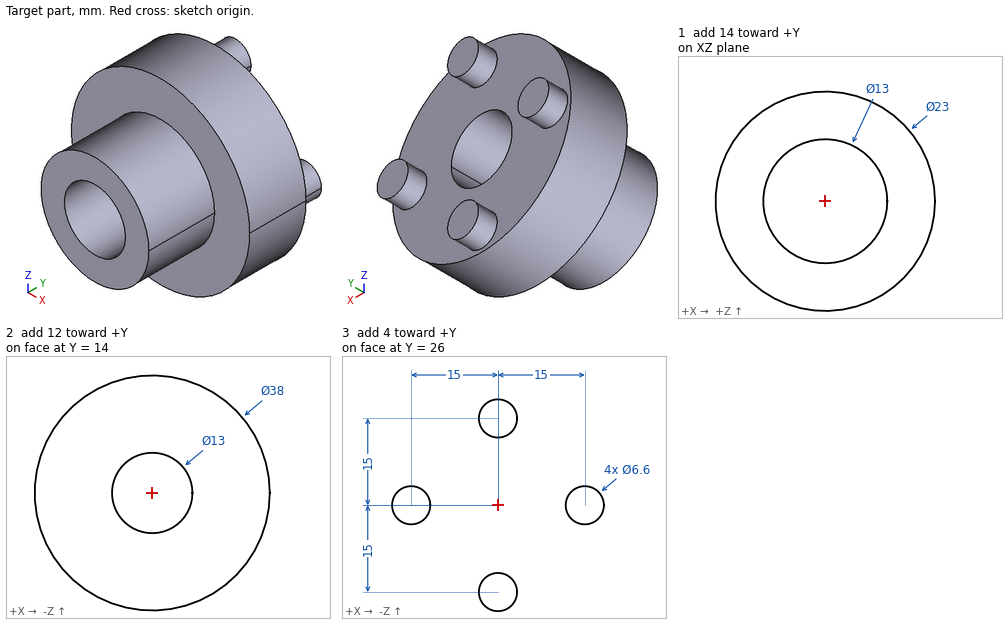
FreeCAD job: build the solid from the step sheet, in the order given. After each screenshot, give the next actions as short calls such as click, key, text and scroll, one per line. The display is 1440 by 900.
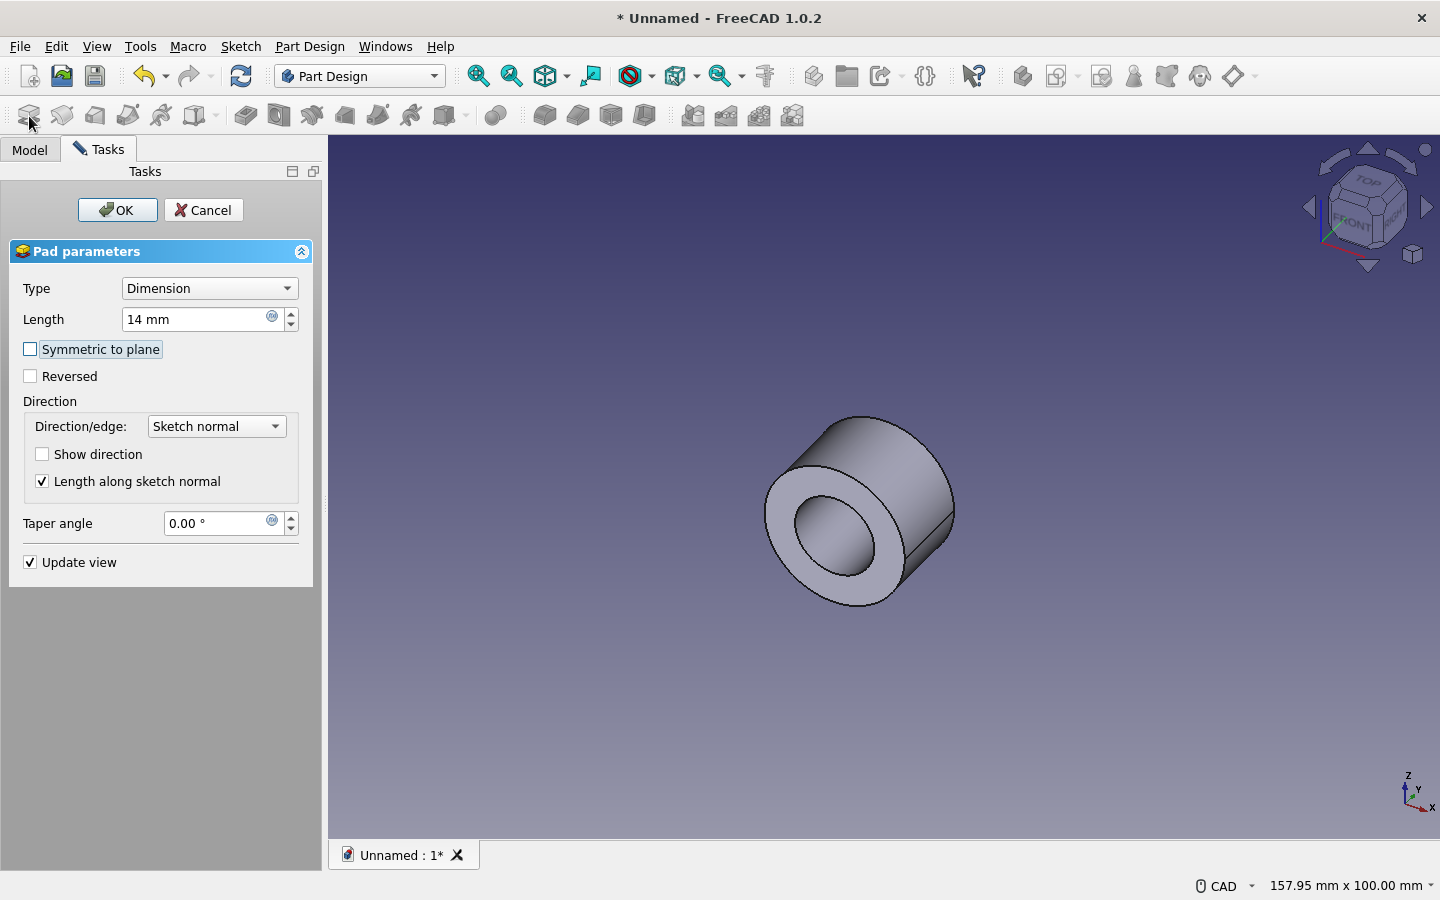
click(31, 376)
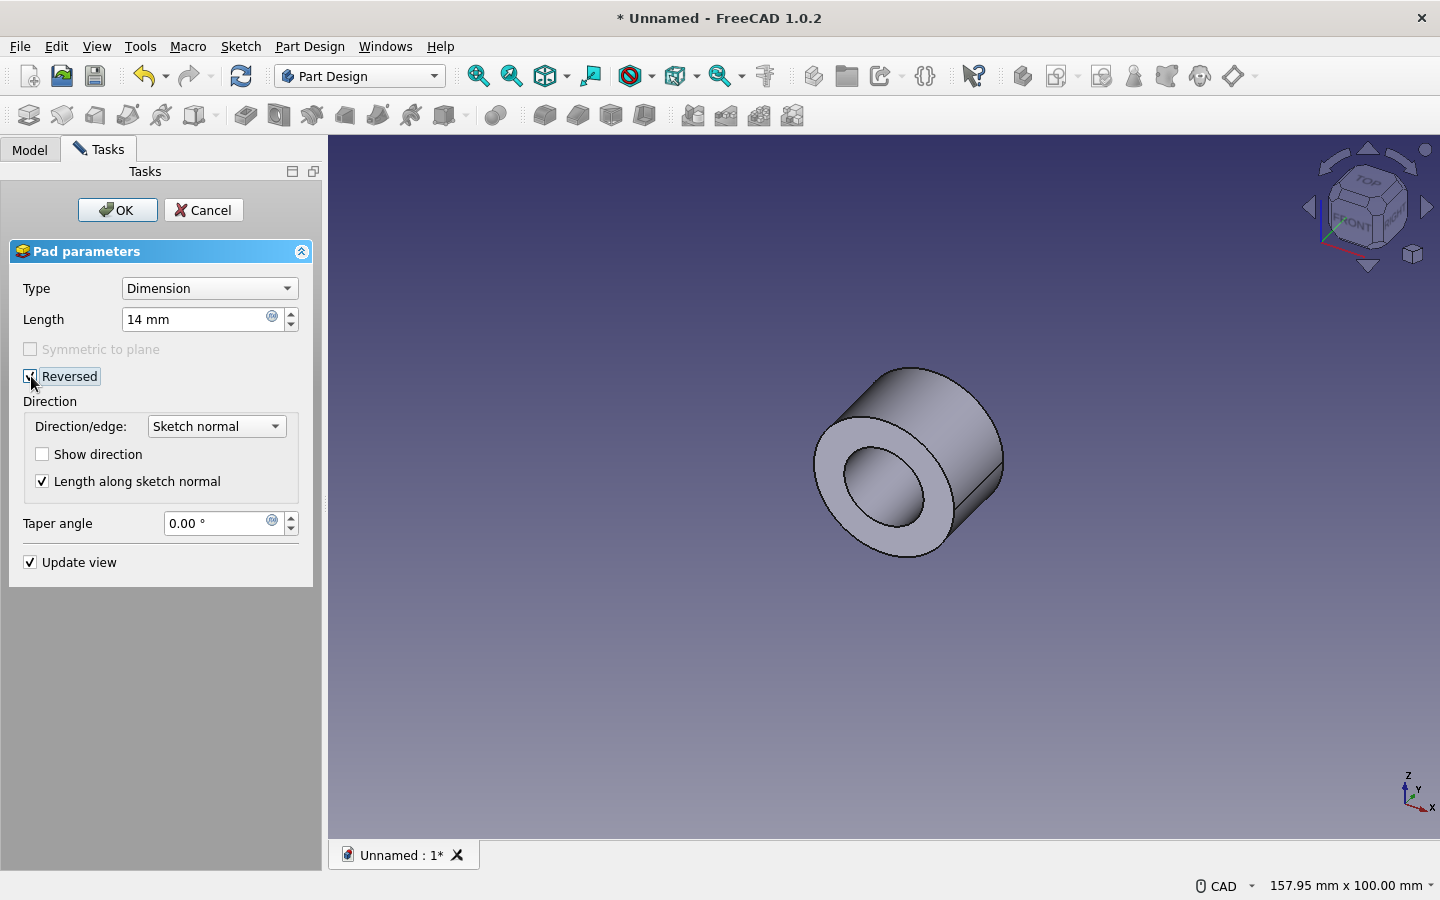
click(118, 210)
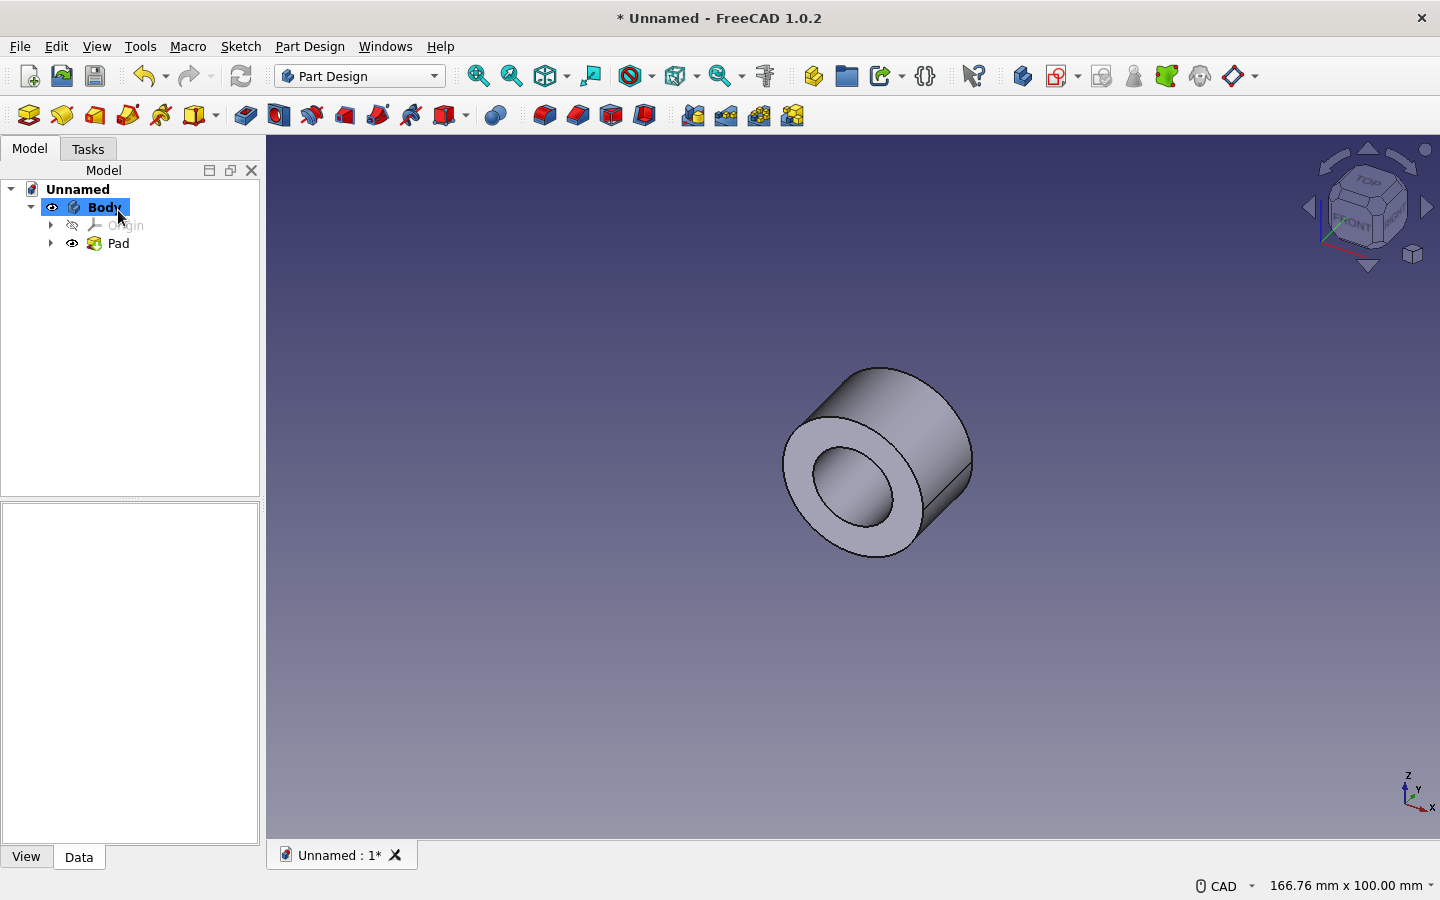
key(v)
key(f)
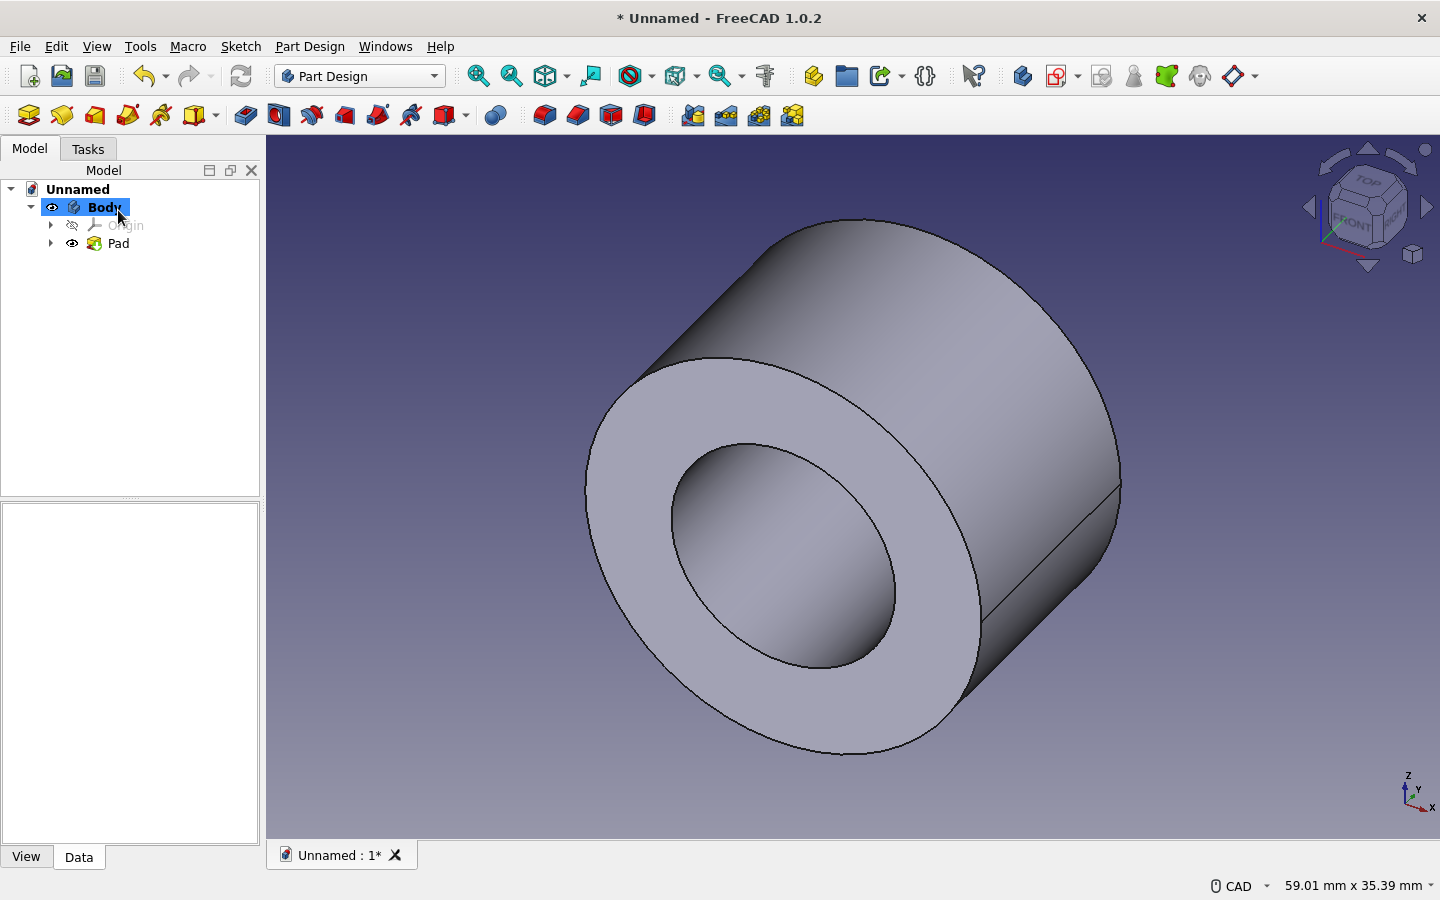
key(4)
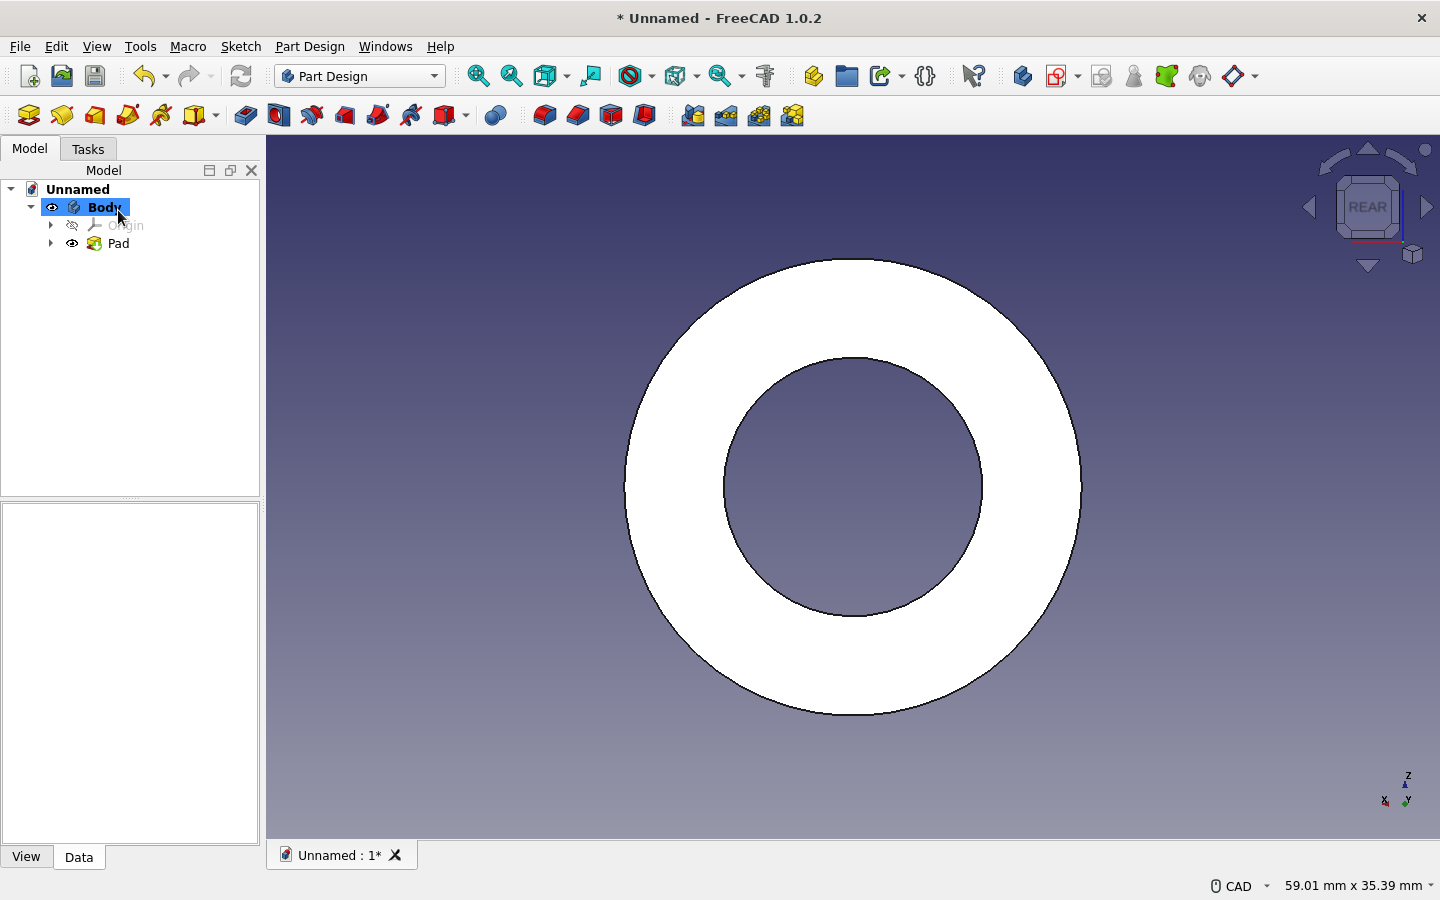
click(722, 617)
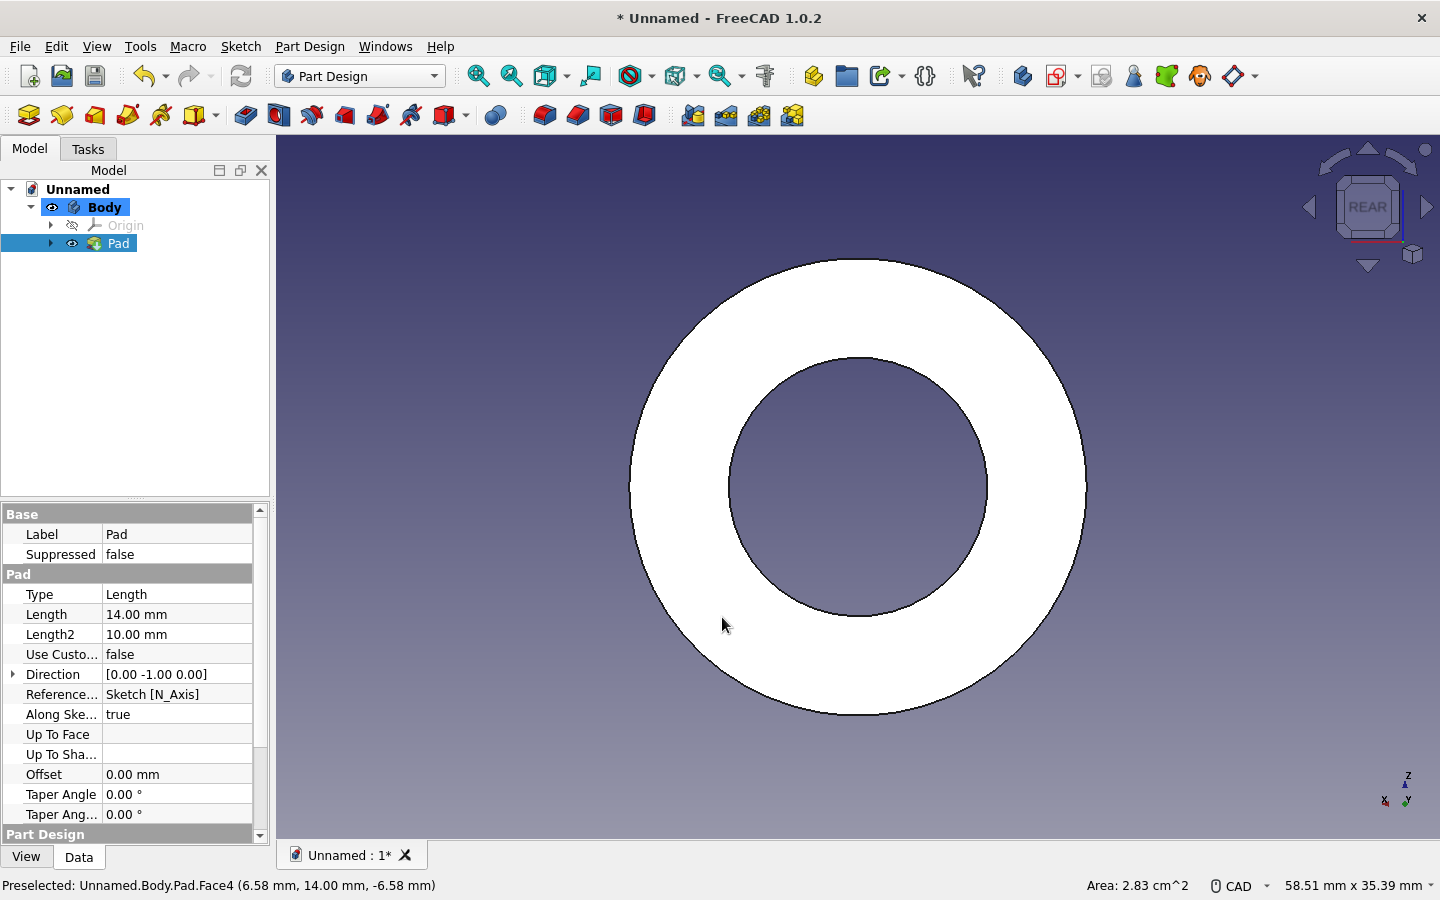
click(1056, 76)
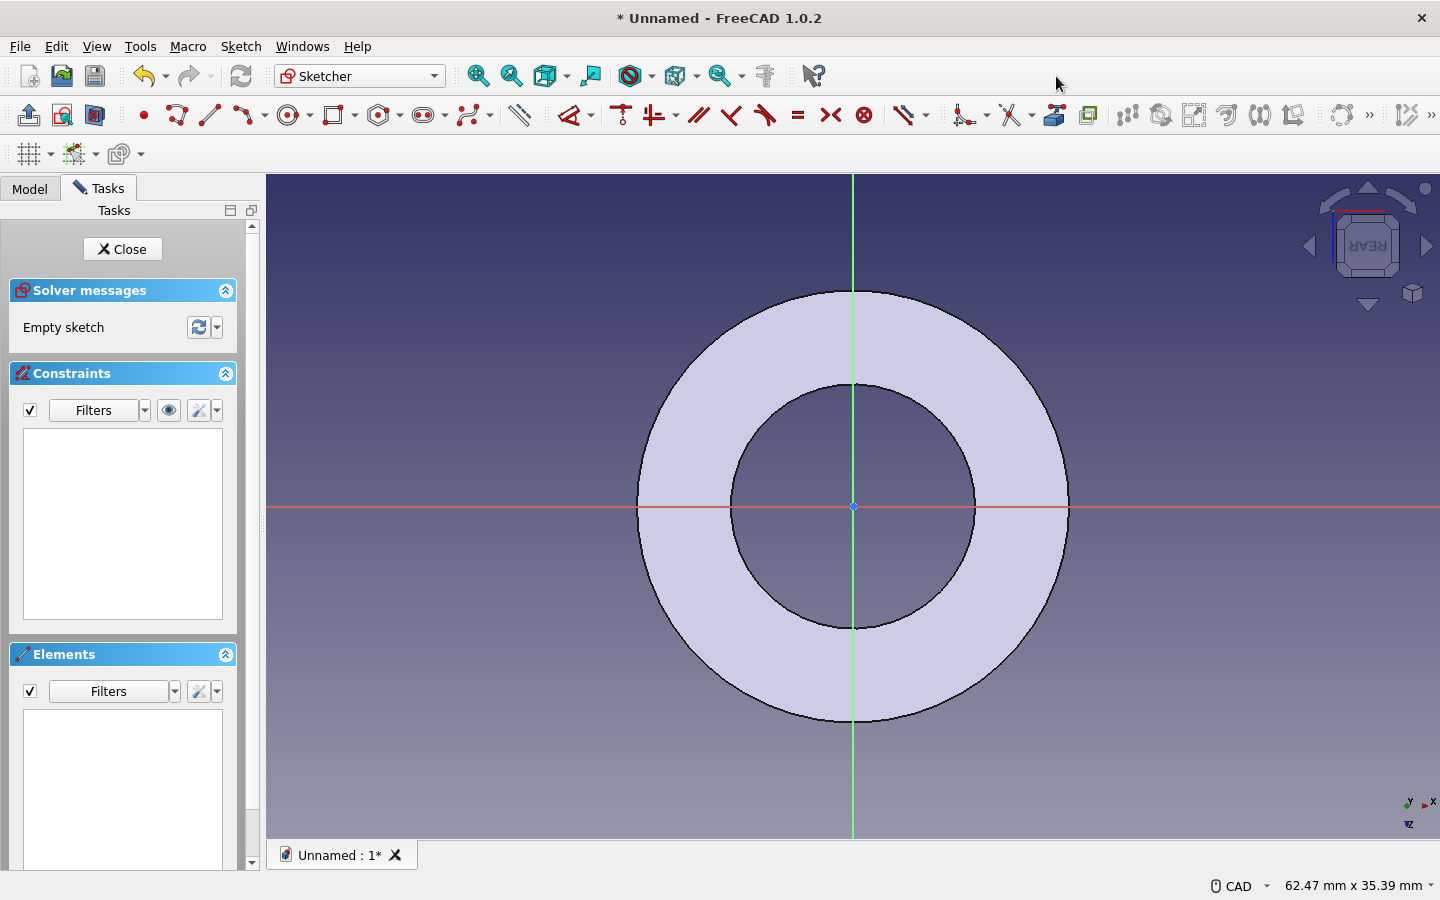
scroll(701, 506, down, 3)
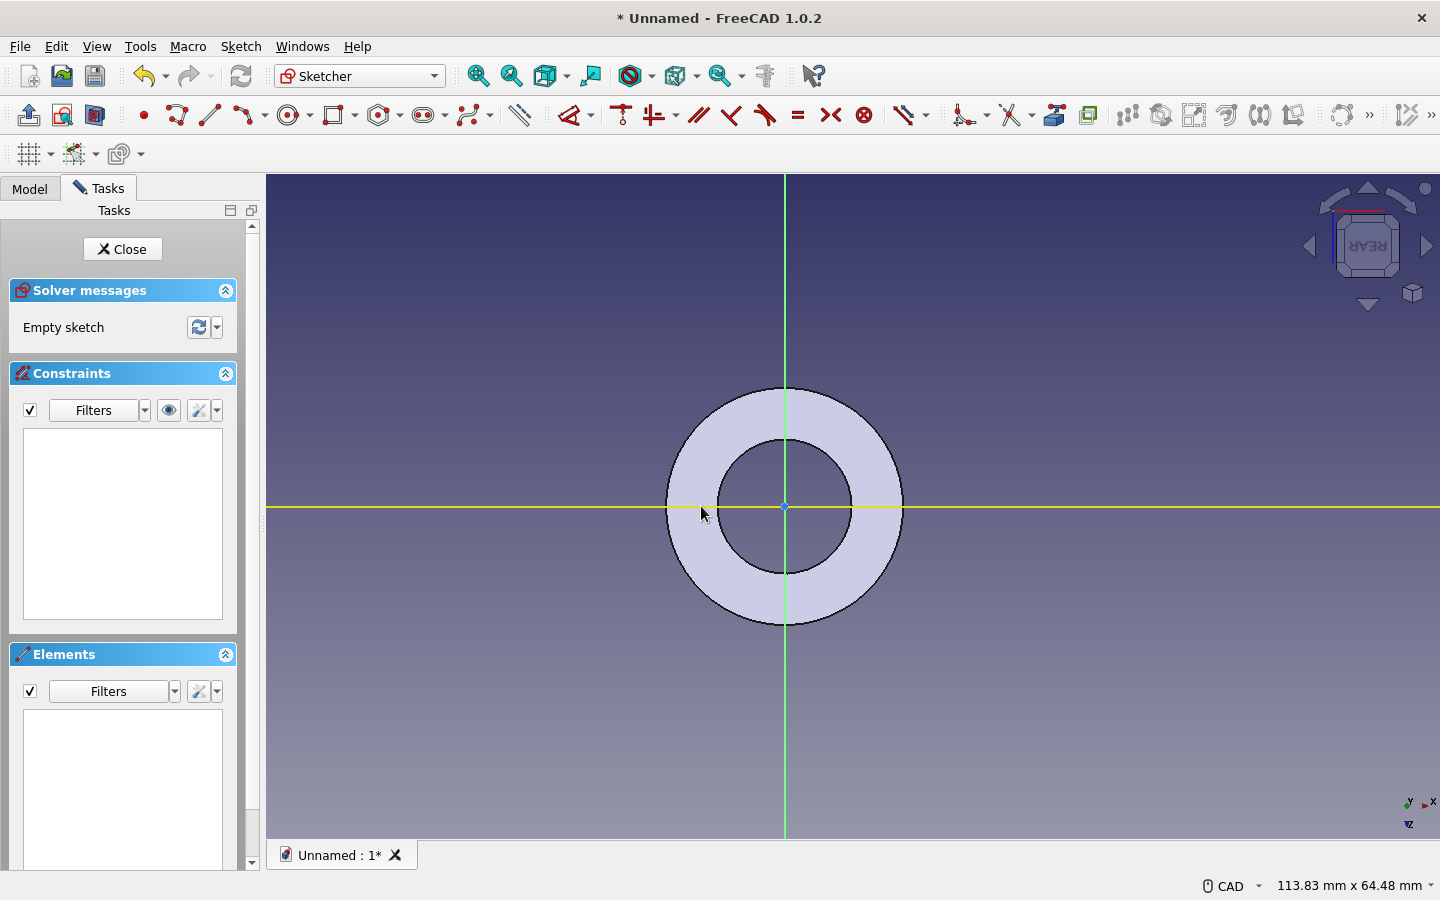
key(g)
key(c)